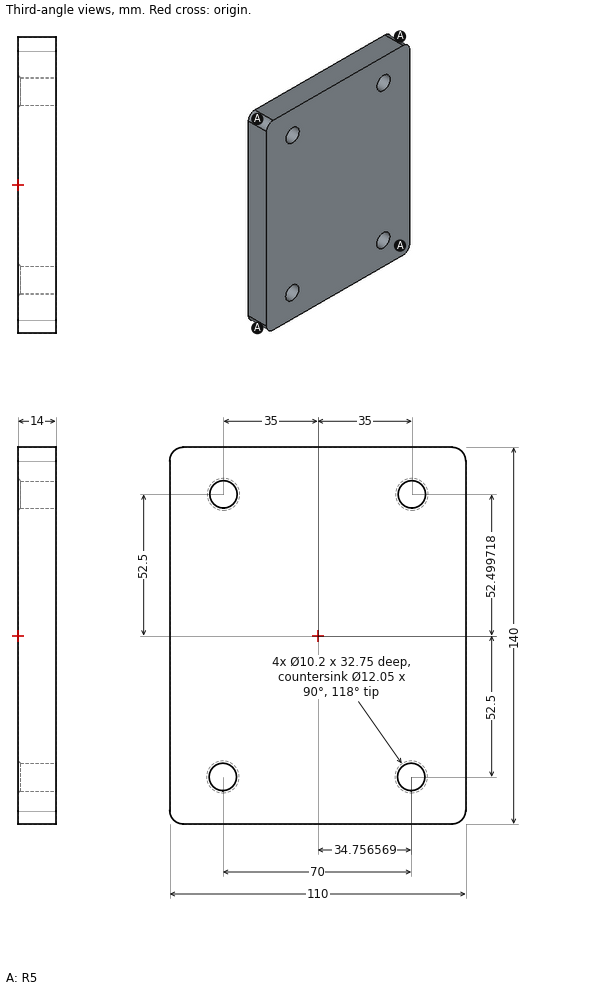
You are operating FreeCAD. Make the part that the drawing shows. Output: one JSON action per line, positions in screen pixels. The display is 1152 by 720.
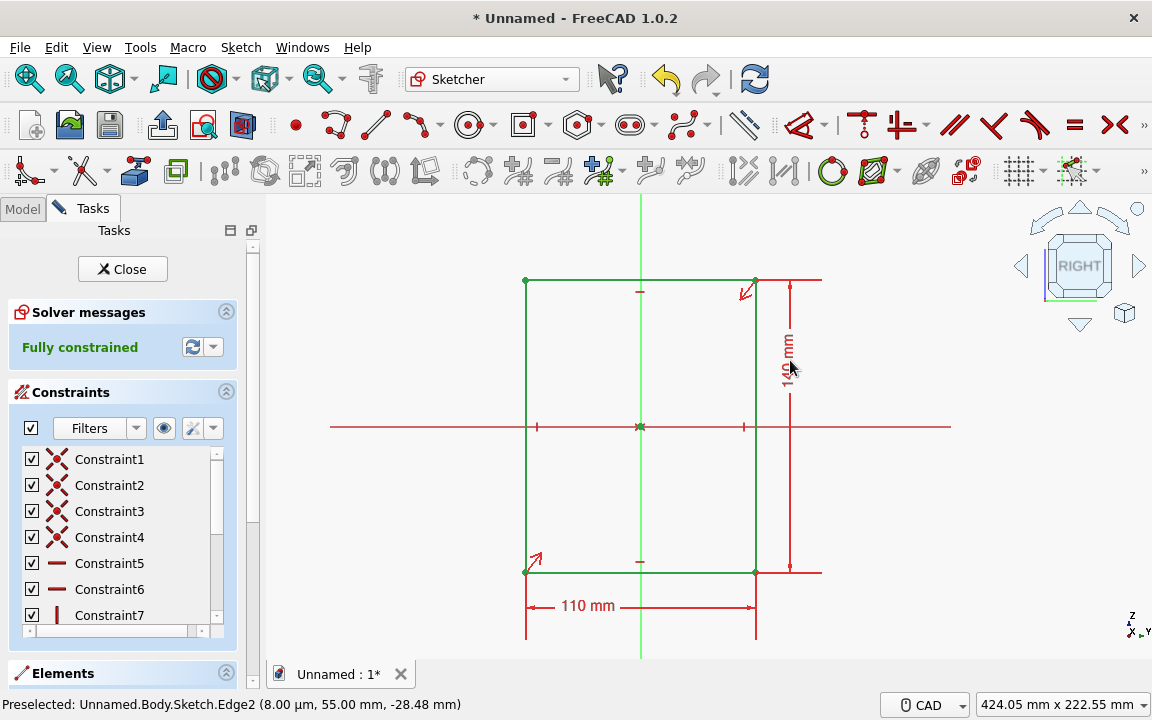
{"action": "left_click", "coordinate": [123, 269]}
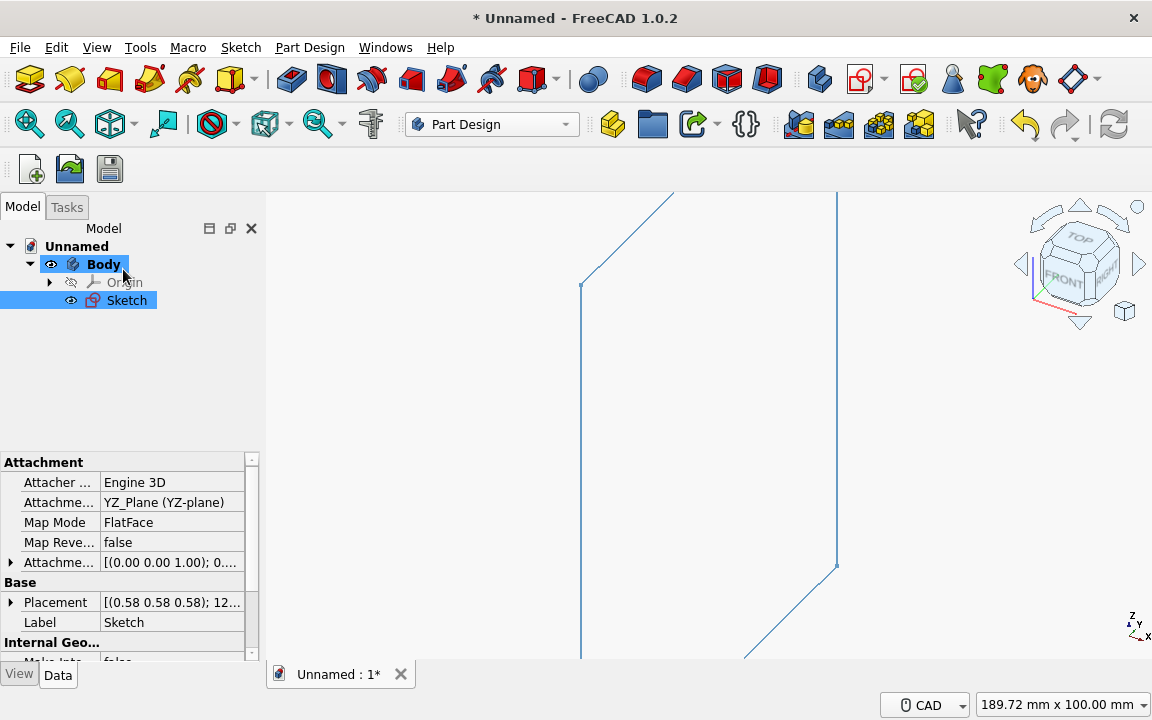
{"action": "left_click", "coordinate": [30, 80]}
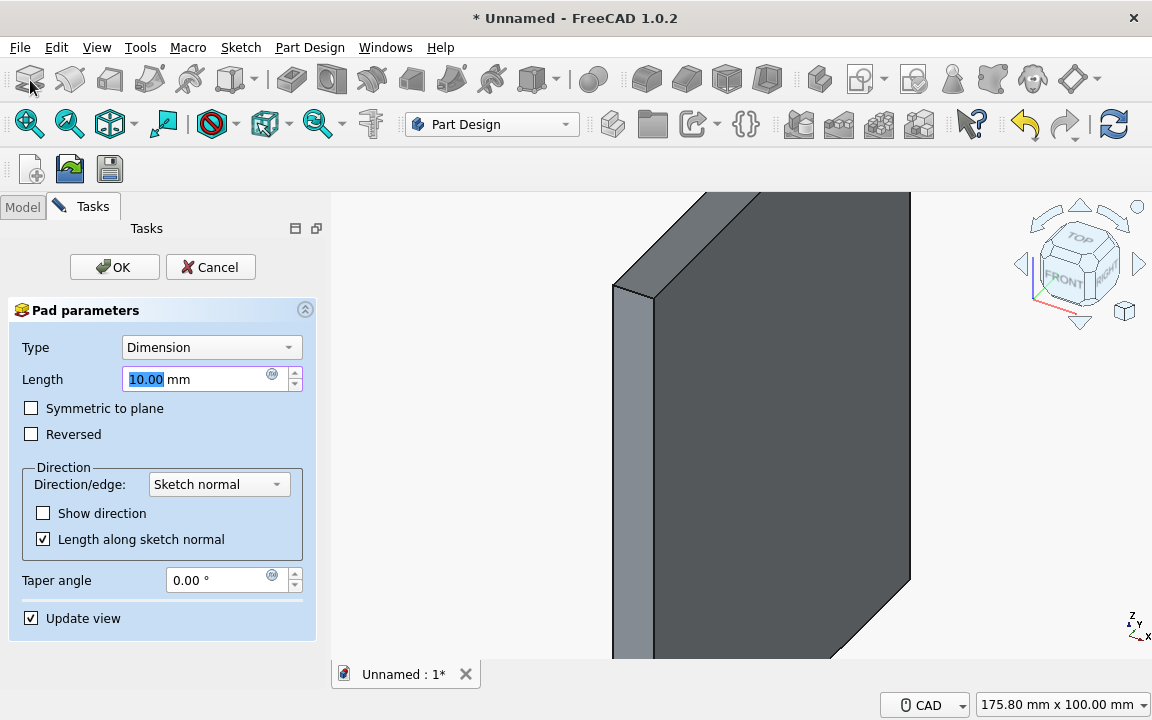
{"action": "type", "text": "14"}
{"action": "key", "text": "Tab"}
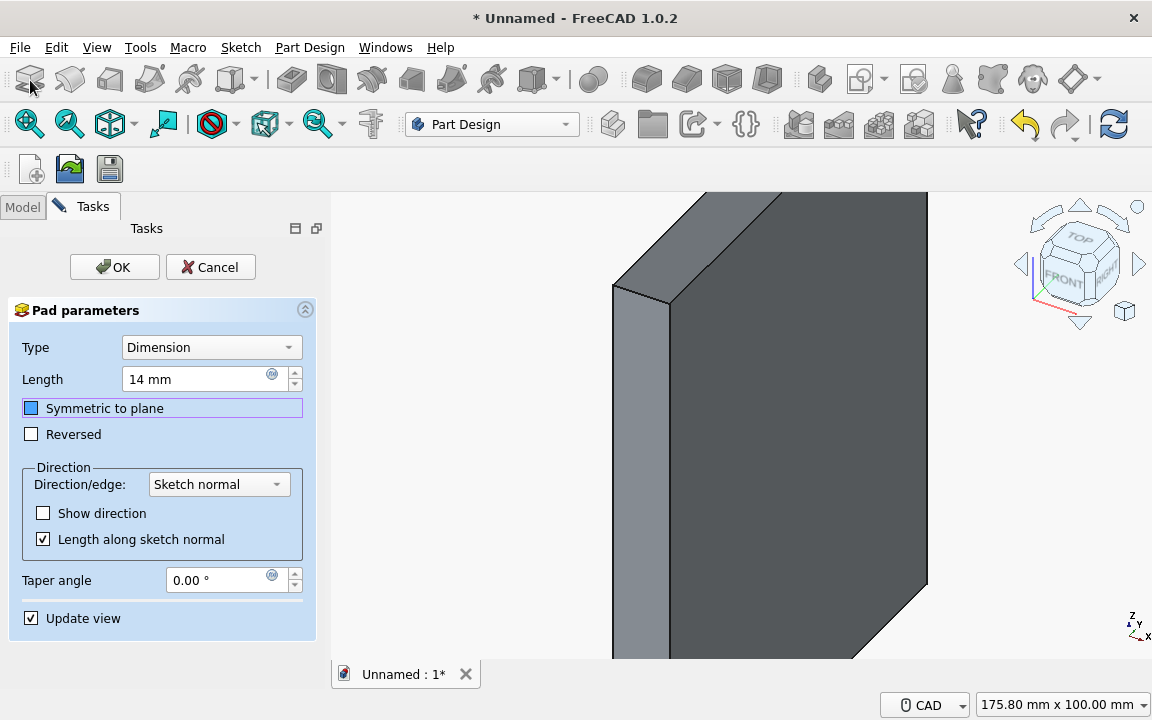
{"action": "left_click", "coordinate": [115, 267]}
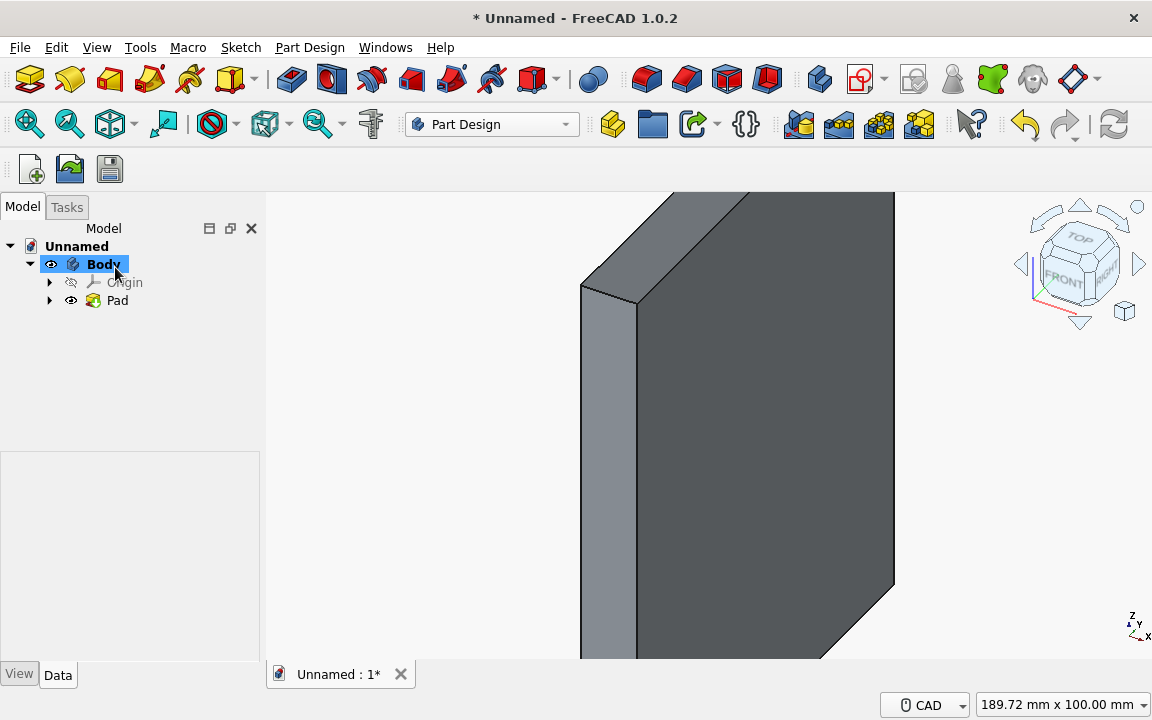
{"action": "left_click", "coordinate": [30, 124]}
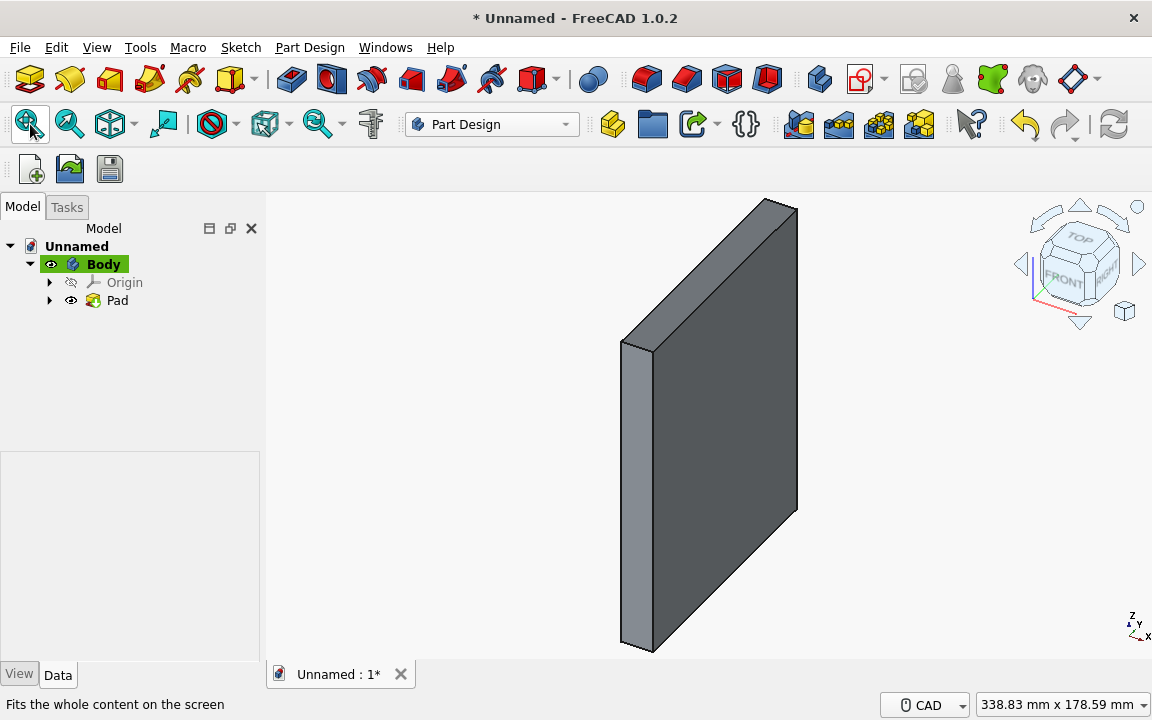
{"action": "left_click", "coordinate": [637, 346]}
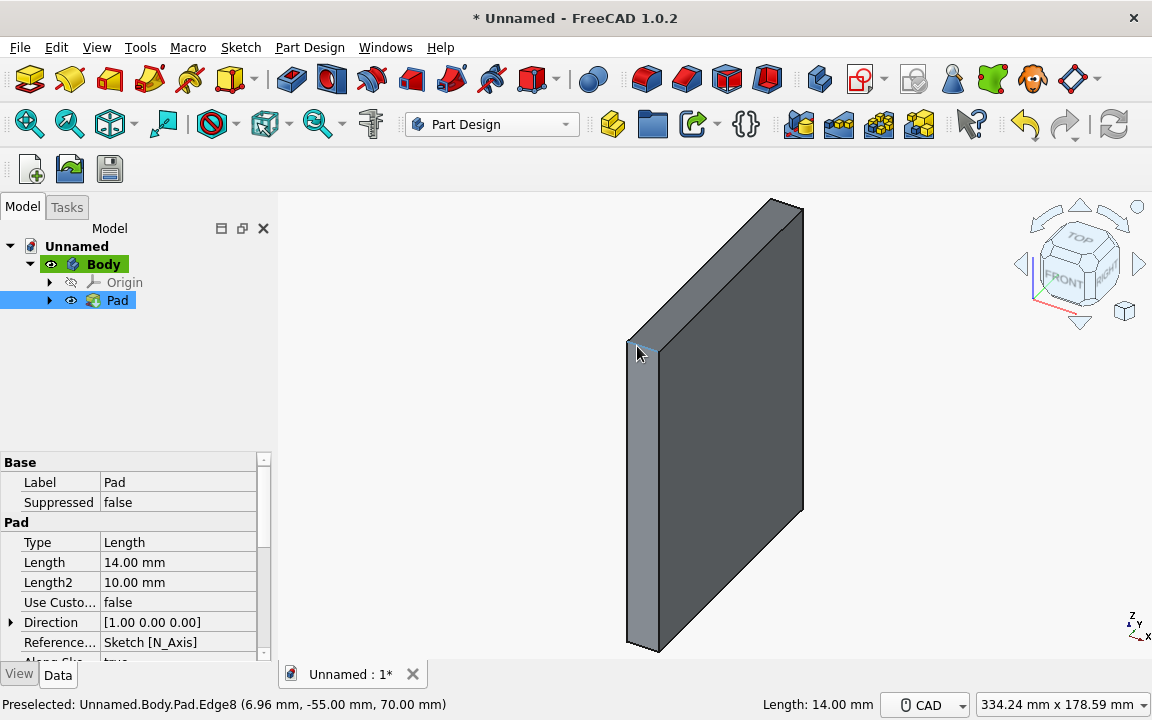
{"action": "key", "text": "0"}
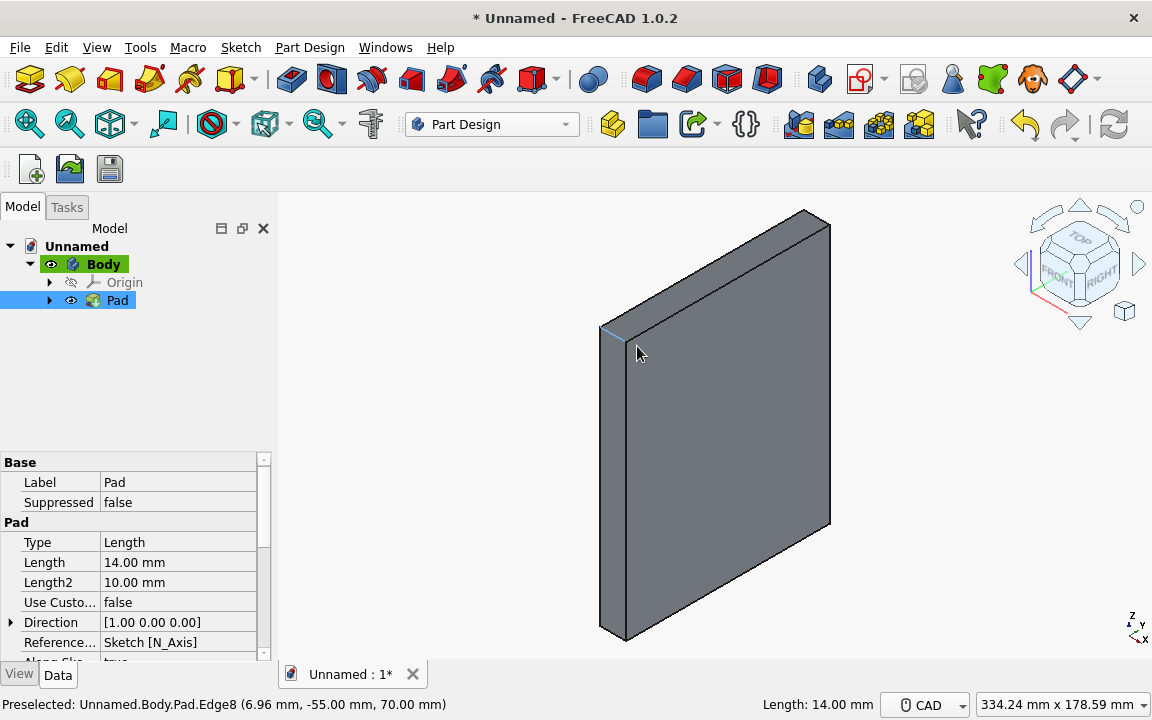
{"action": "key", "text": "2"}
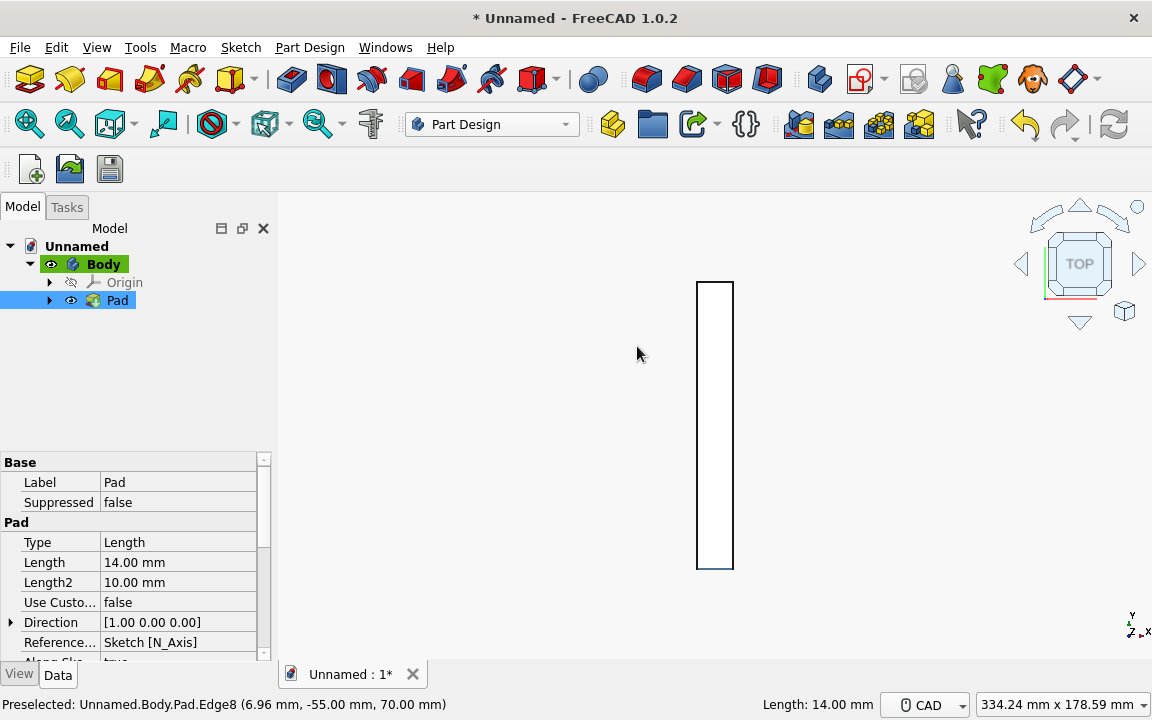
{"action": "left_click", "coordinate": [715, 281], "text": "ctrl"}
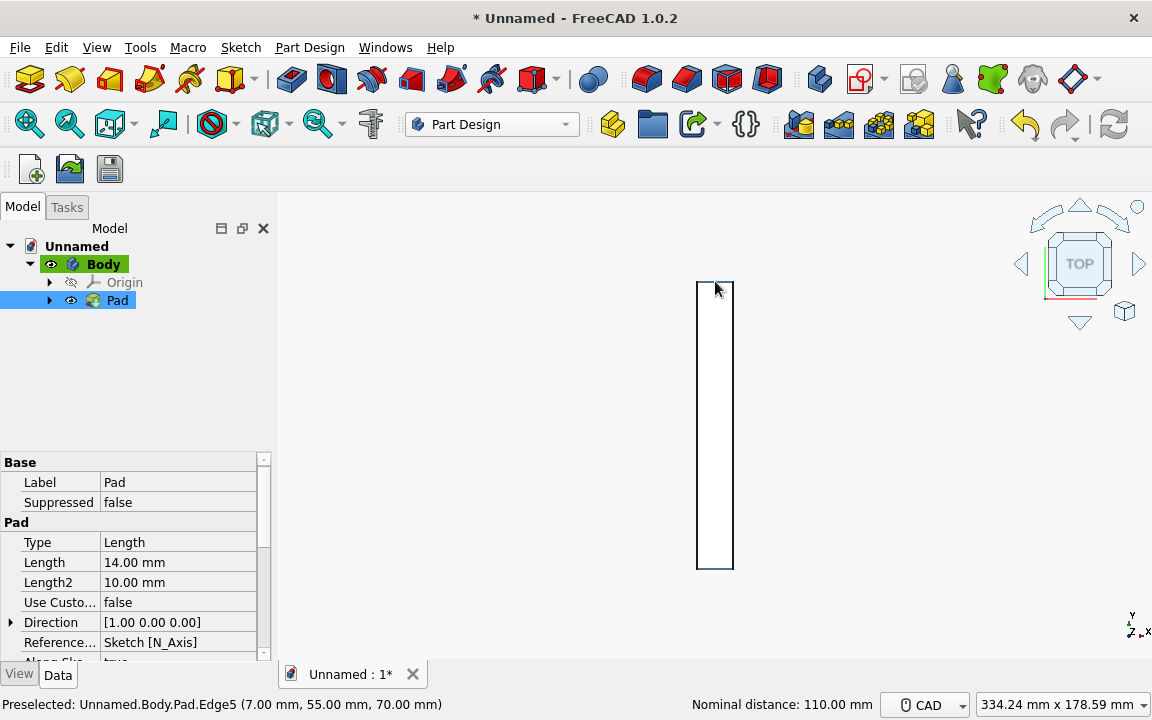
{"action": "key", "text": "1"}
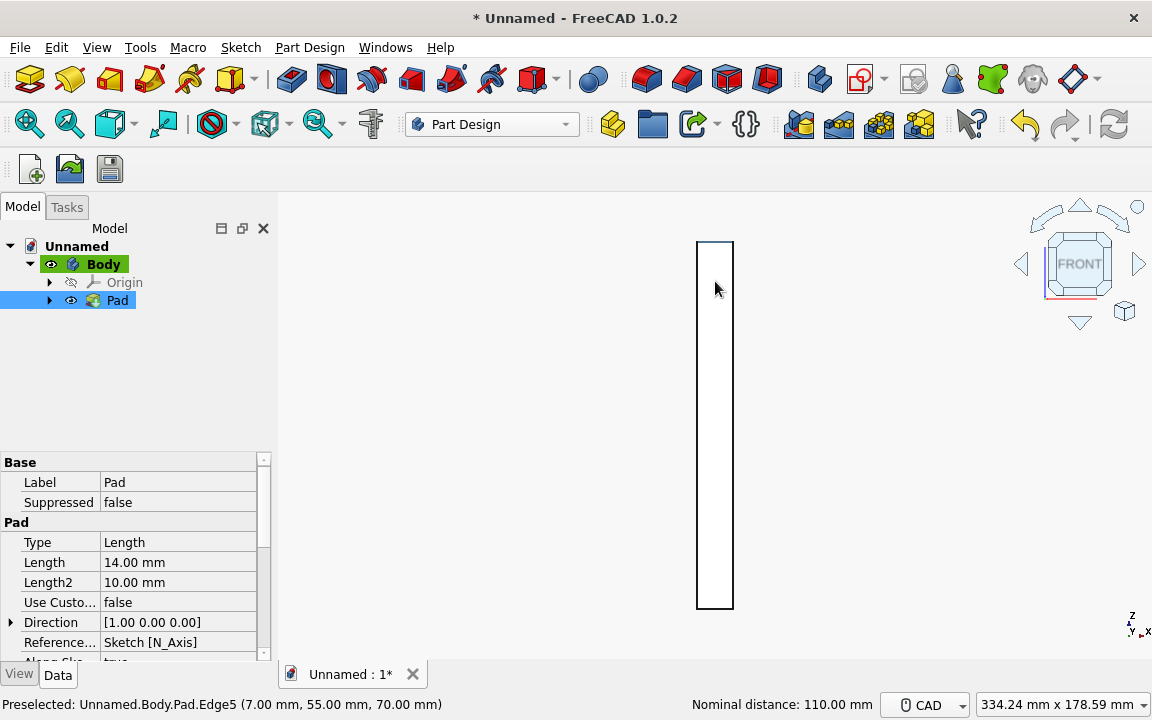
{"action": "left_click", "coordinate": [715, 608], "text": "ctrl"}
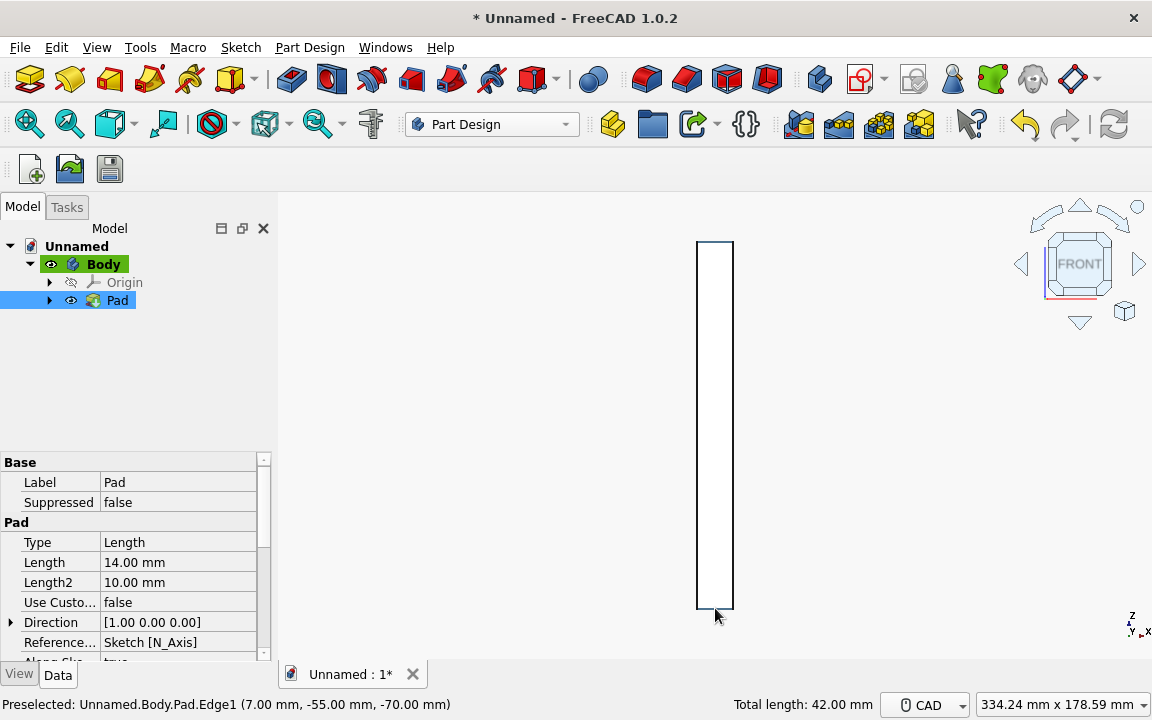
{"action": "key", "text": "3"}